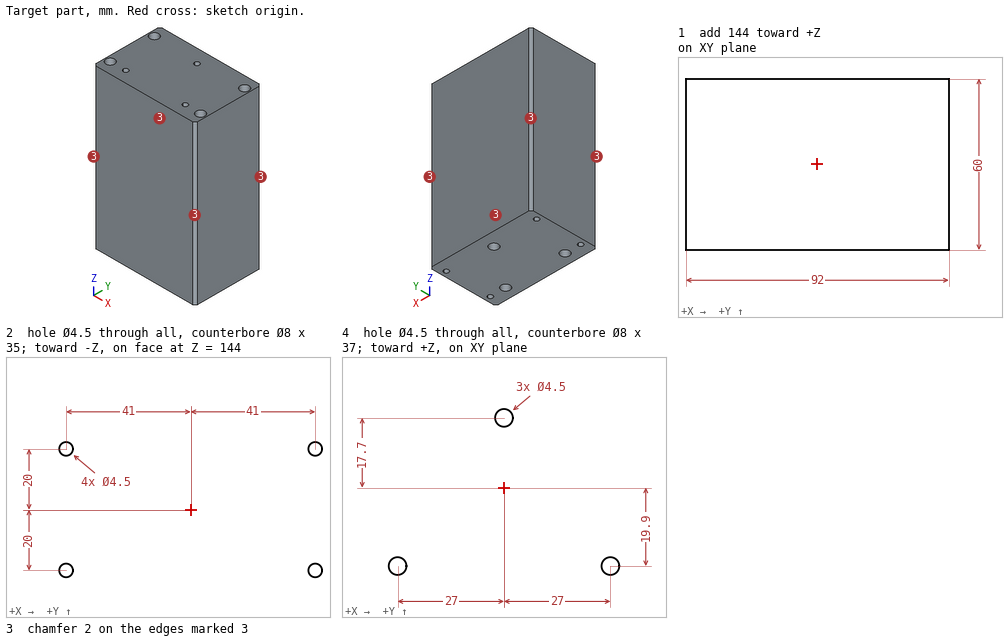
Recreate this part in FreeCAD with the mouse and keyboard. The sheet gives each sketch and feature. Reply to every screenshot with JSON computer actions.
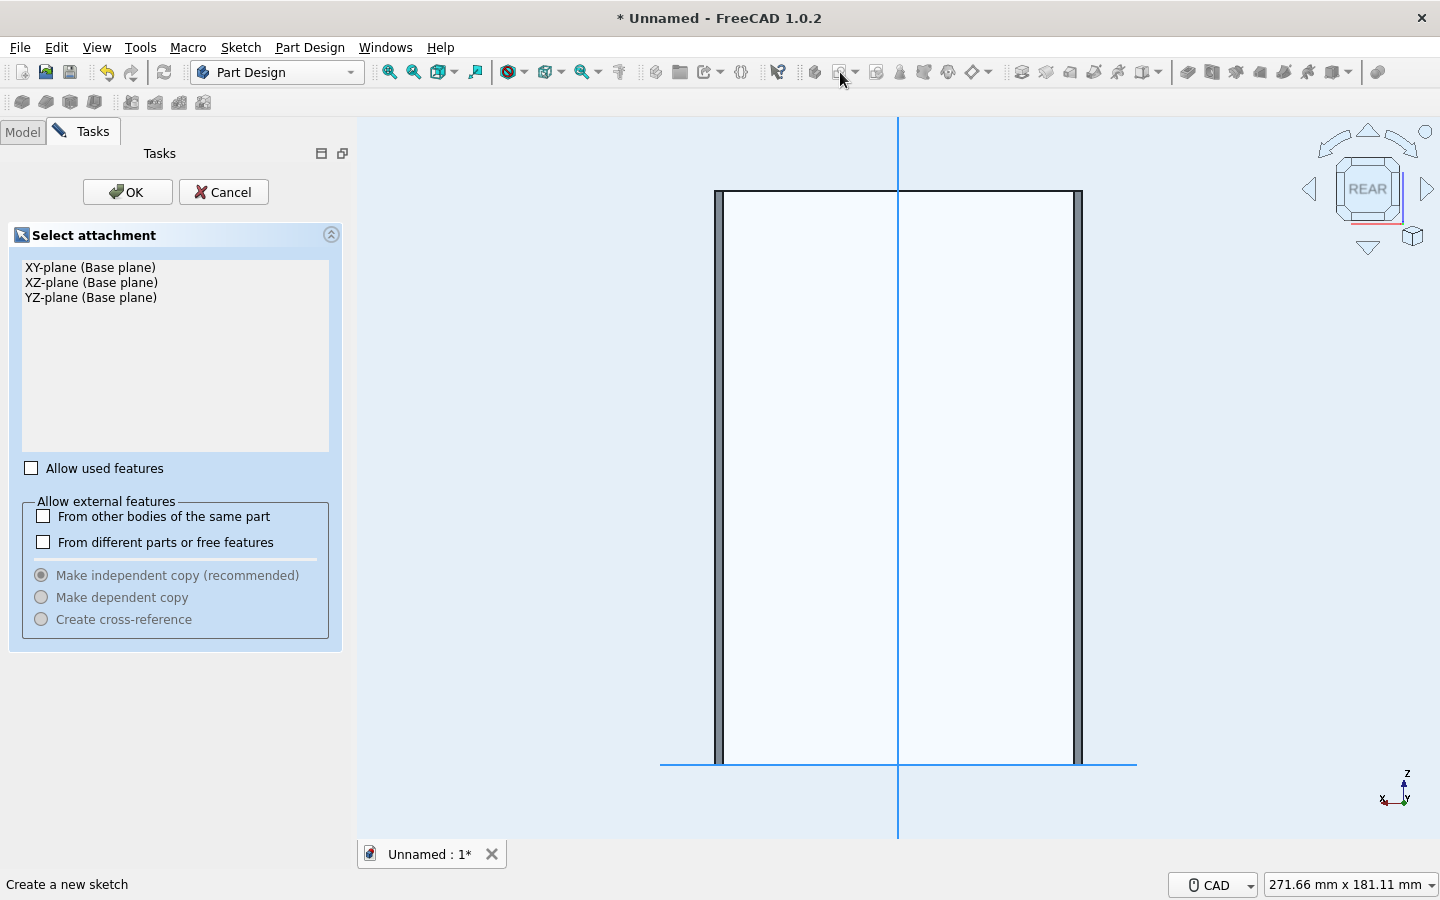
{"action": "left_click", "coordinate": [82, 268]}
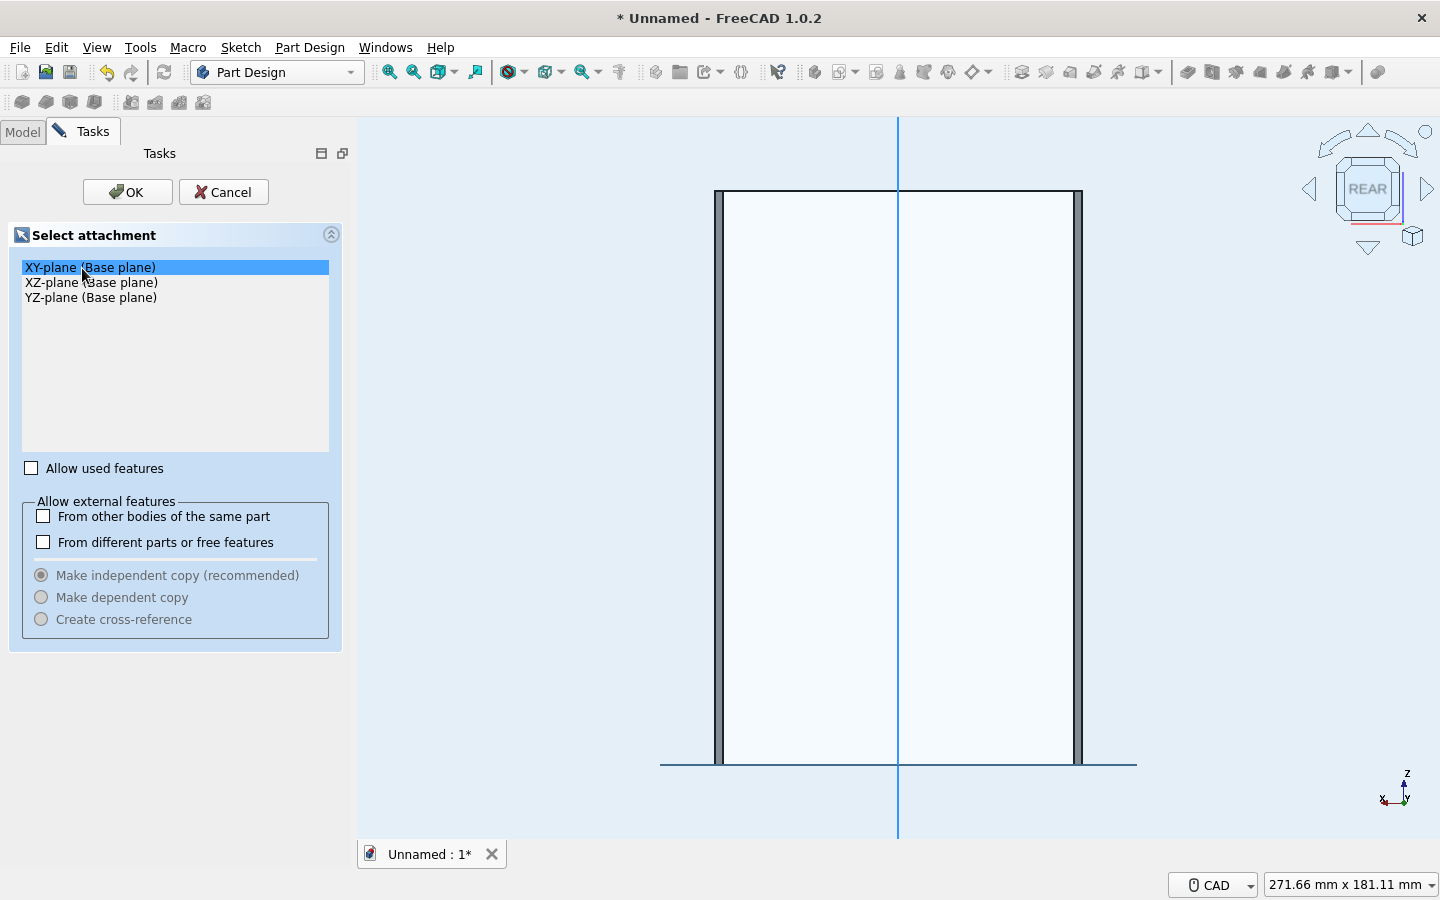
{"action": "left_click", "coordinate": [128, 192]}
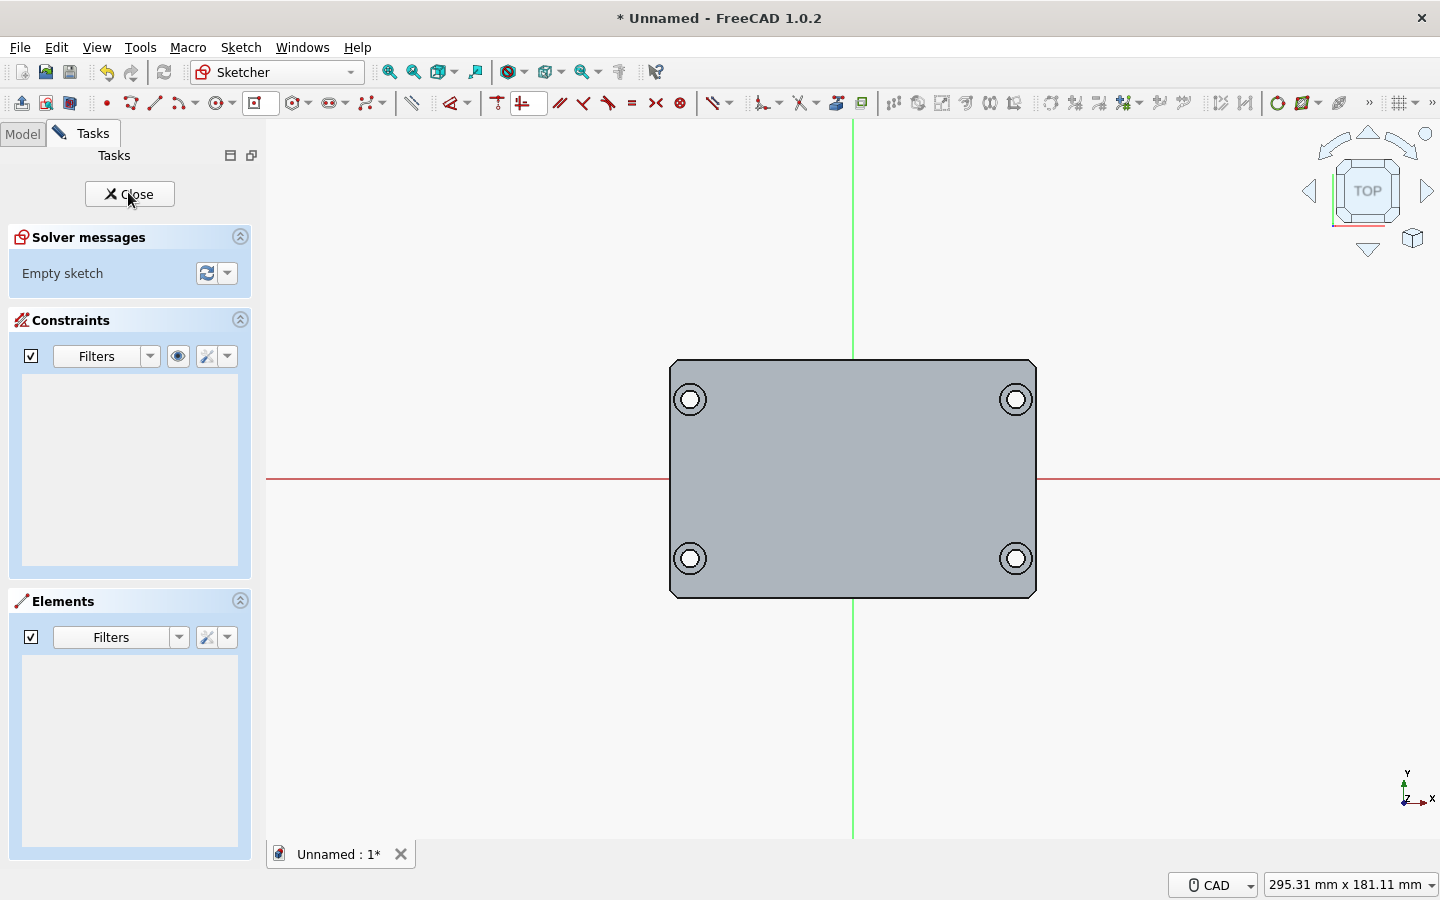
{"action": "left_click", "coordinate": [70, 104]}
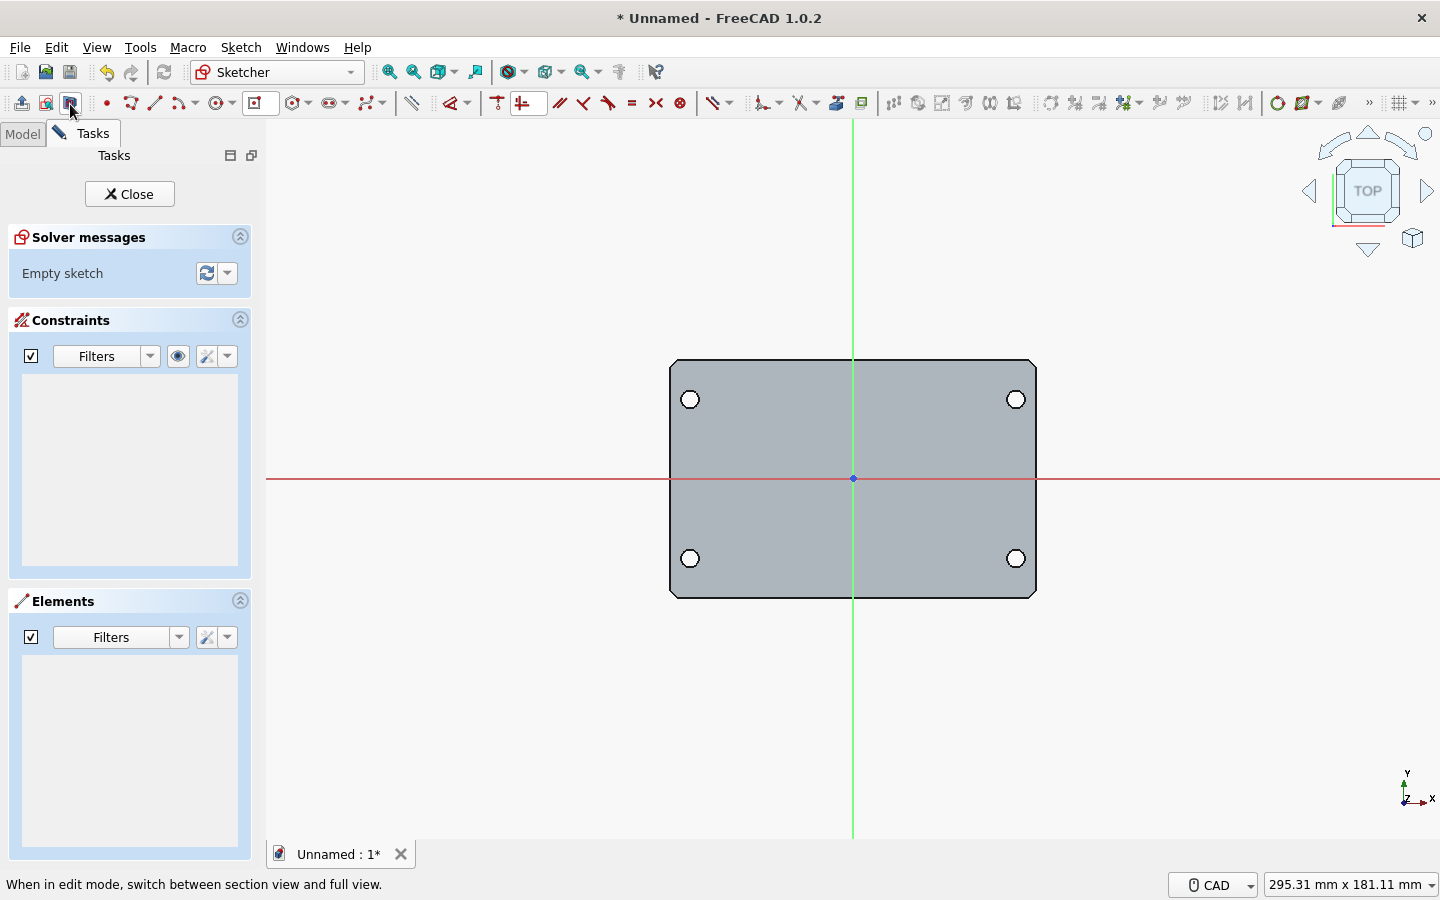
{"action": "scroll", "coordinate": [893, 486], "scroll_direction": "up", "scroll_amount": 5}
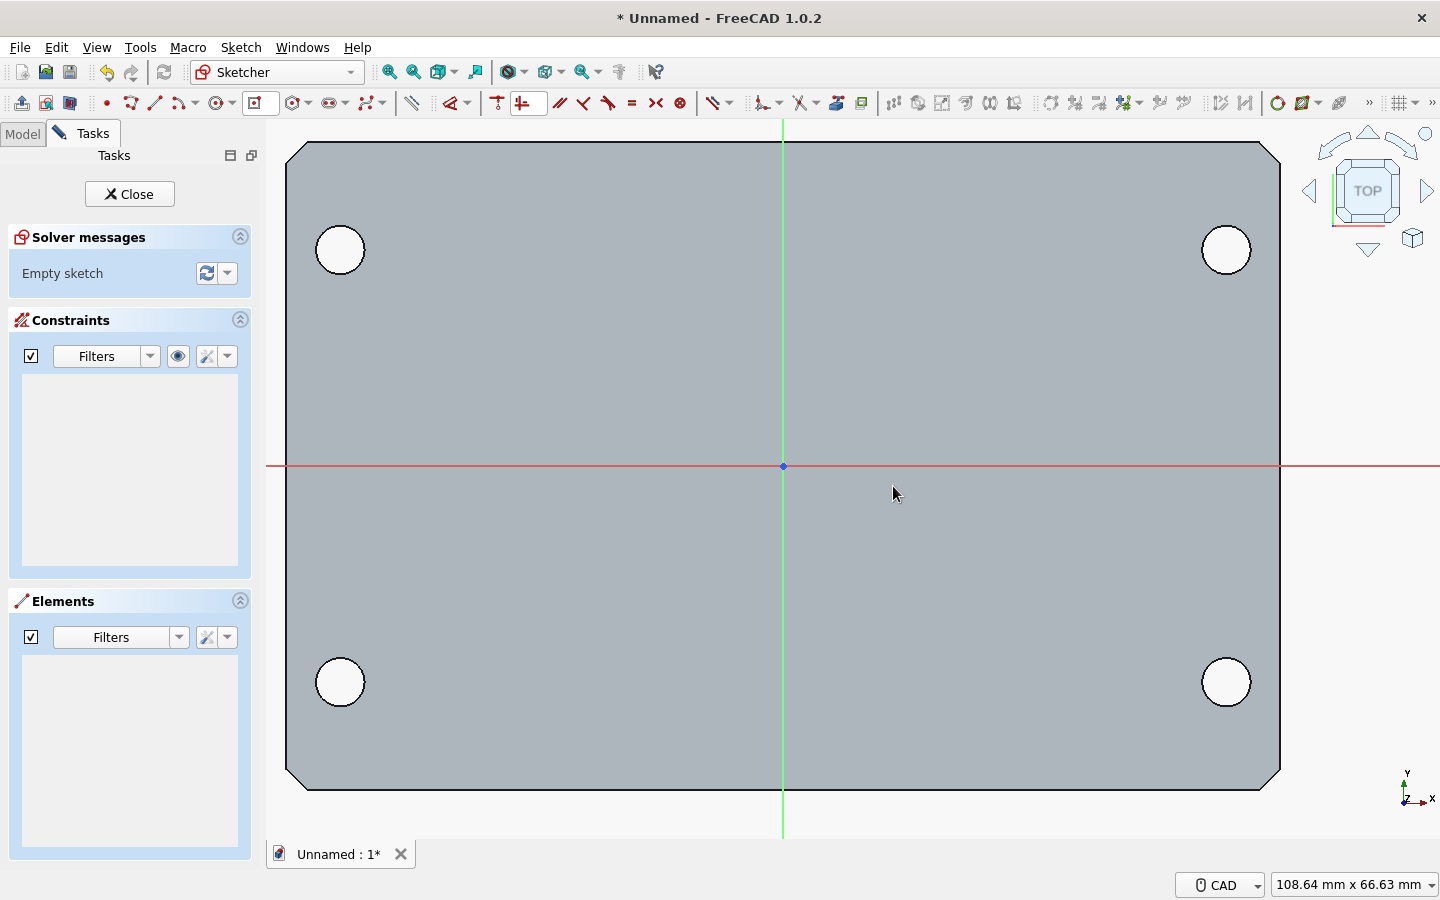
{"action": "left_click", "coordinate": [216, 104]}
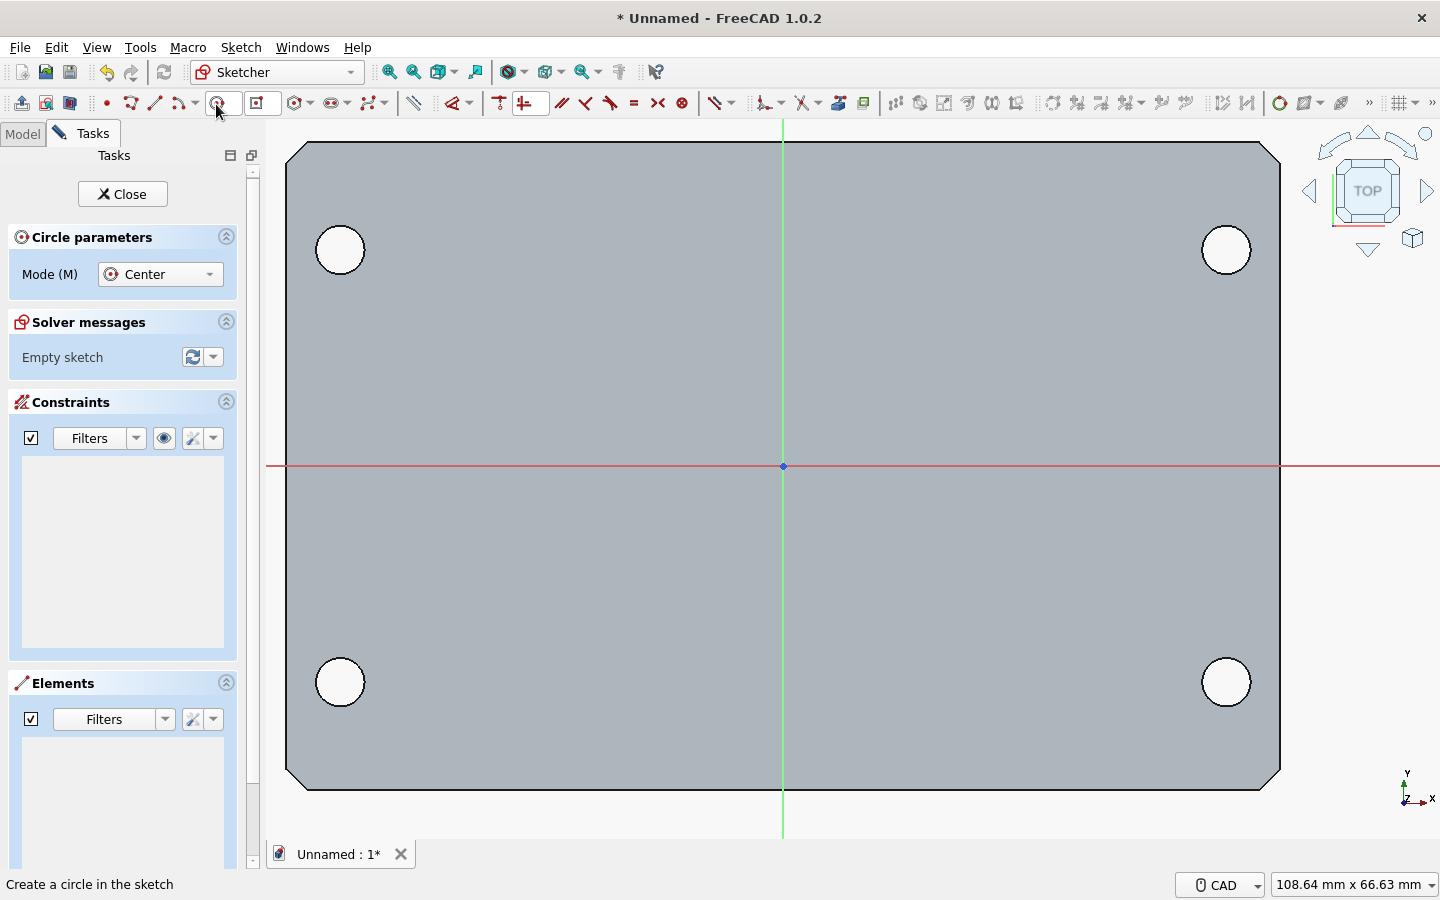
{"action": "left_click", "coordinate": [783, 275]}
{"action": "left_click", "coordinate": [801, 258]}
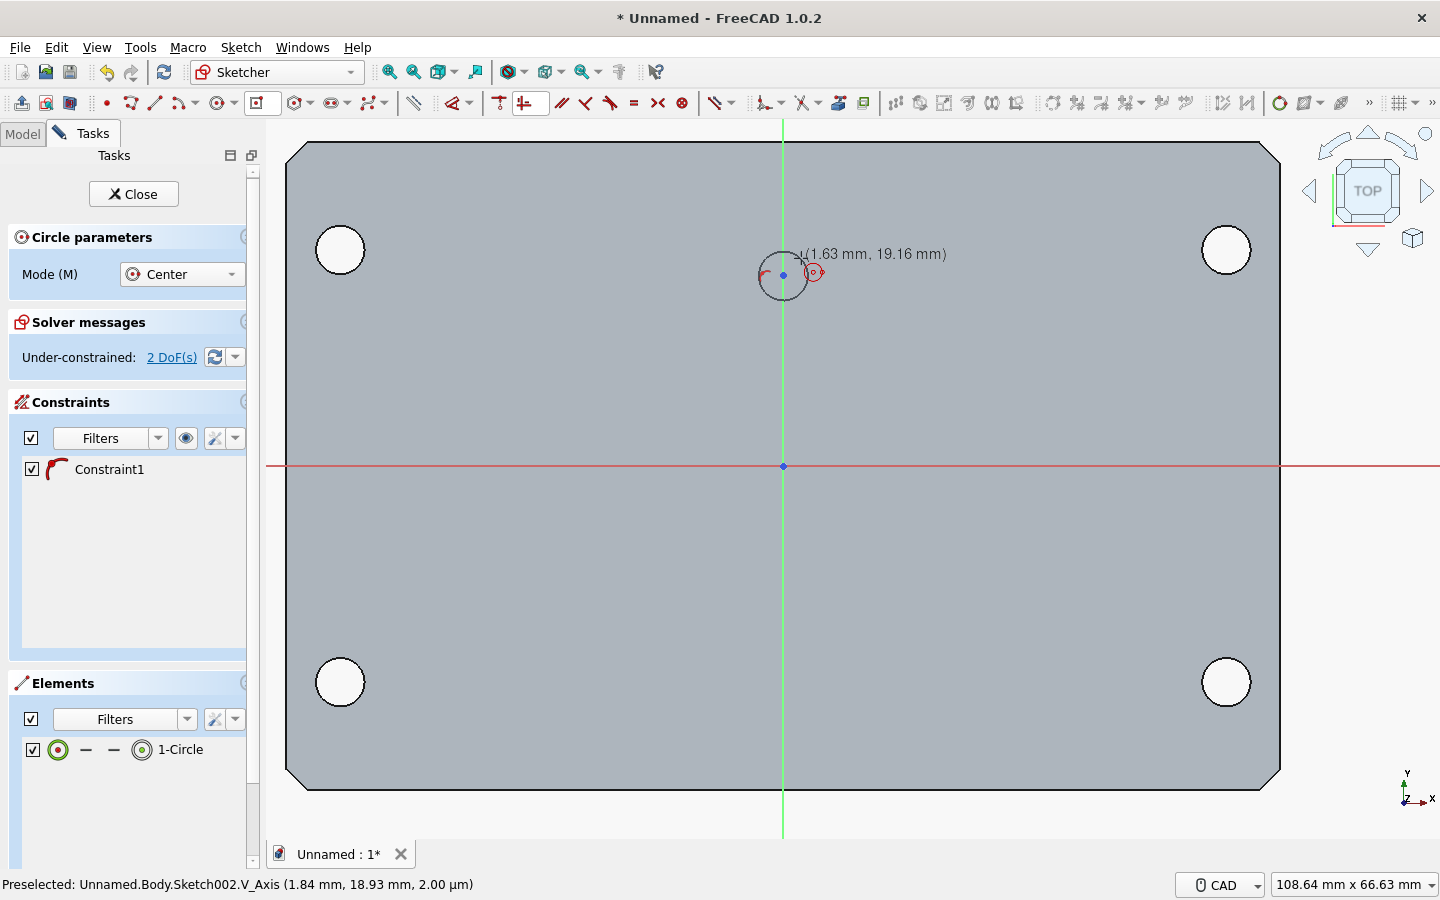
{"action": "left_click", "coordinate": [1075, 681]}
{"action": "left_click", "coordinate": [1092, 664]}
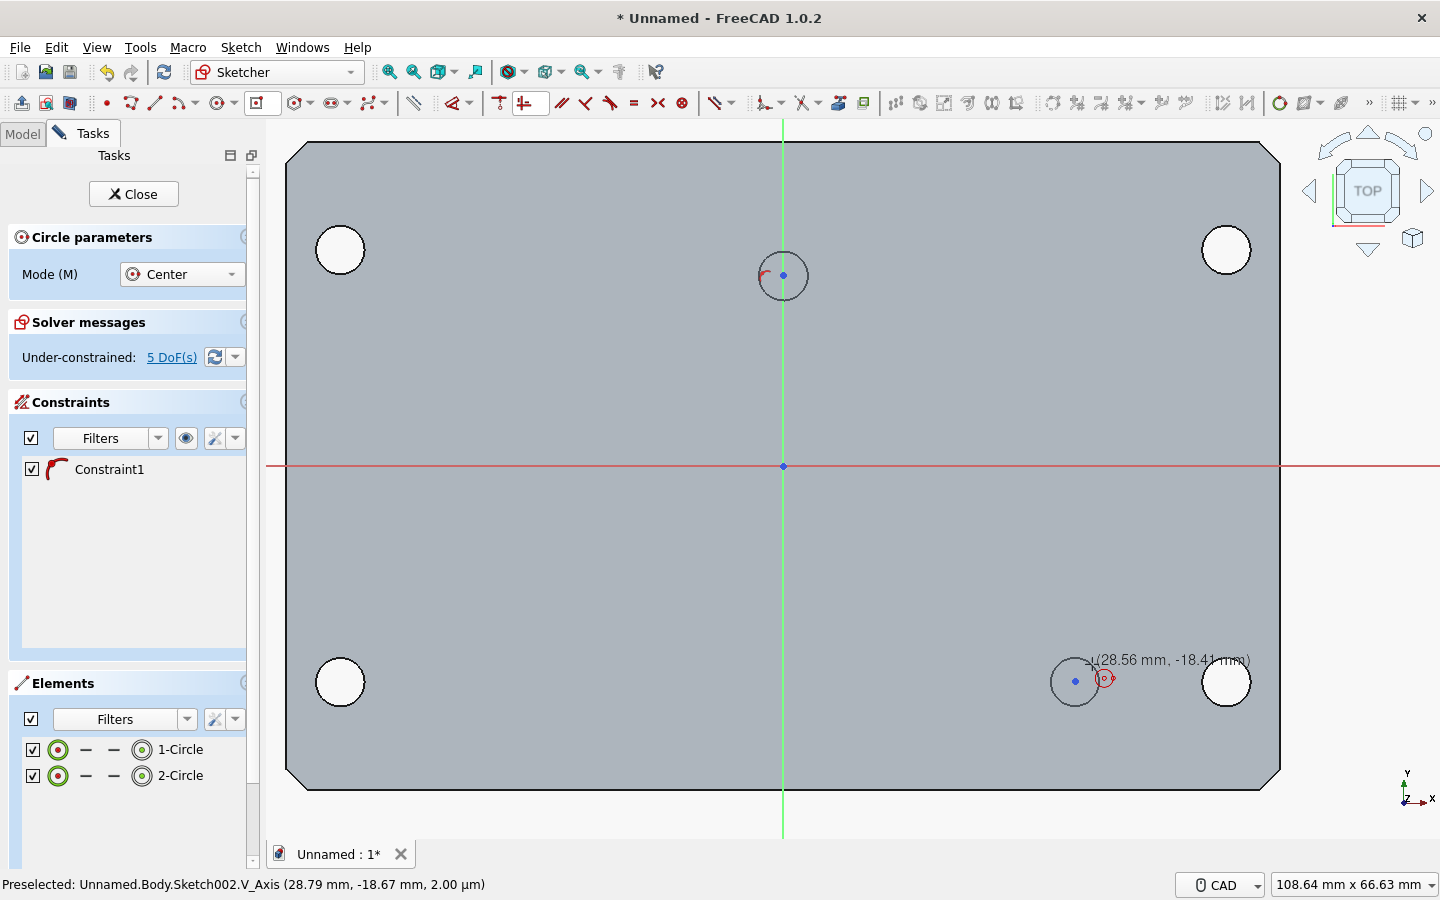
{"action": "left_click", "coordinate": [492, 681]}
{"action": "left_click", "coordinate": [509, 664]}
{"action": "key", "text": "Escape"}